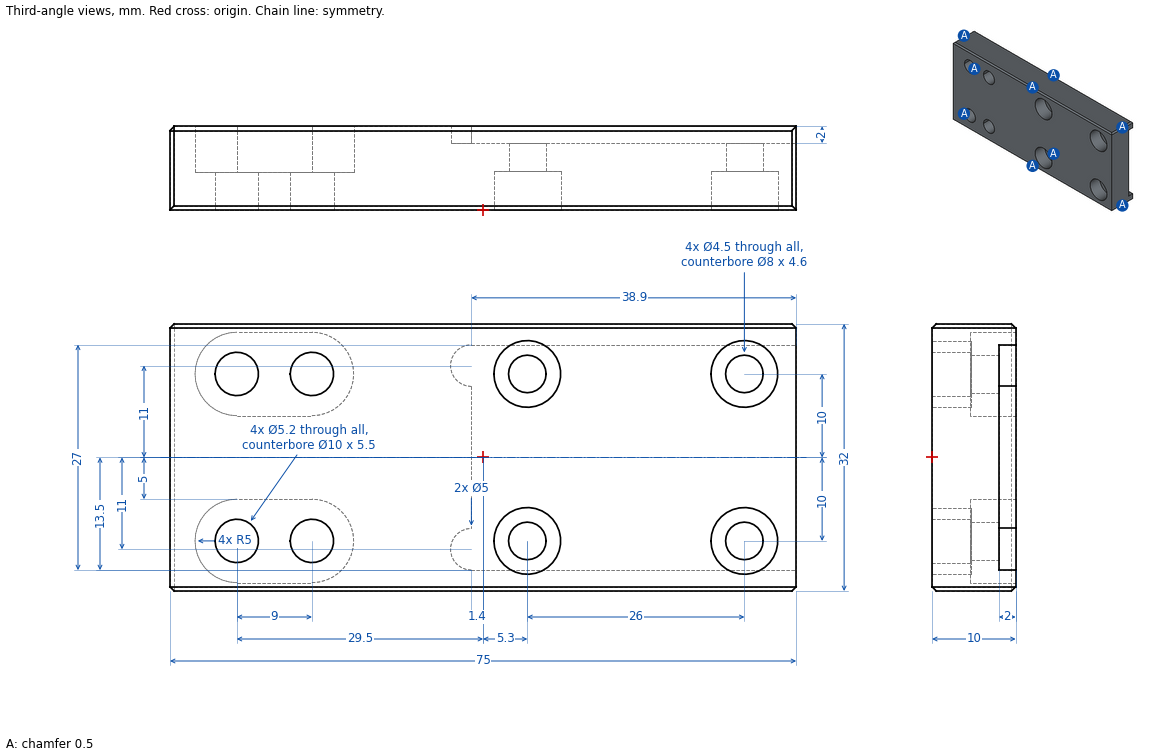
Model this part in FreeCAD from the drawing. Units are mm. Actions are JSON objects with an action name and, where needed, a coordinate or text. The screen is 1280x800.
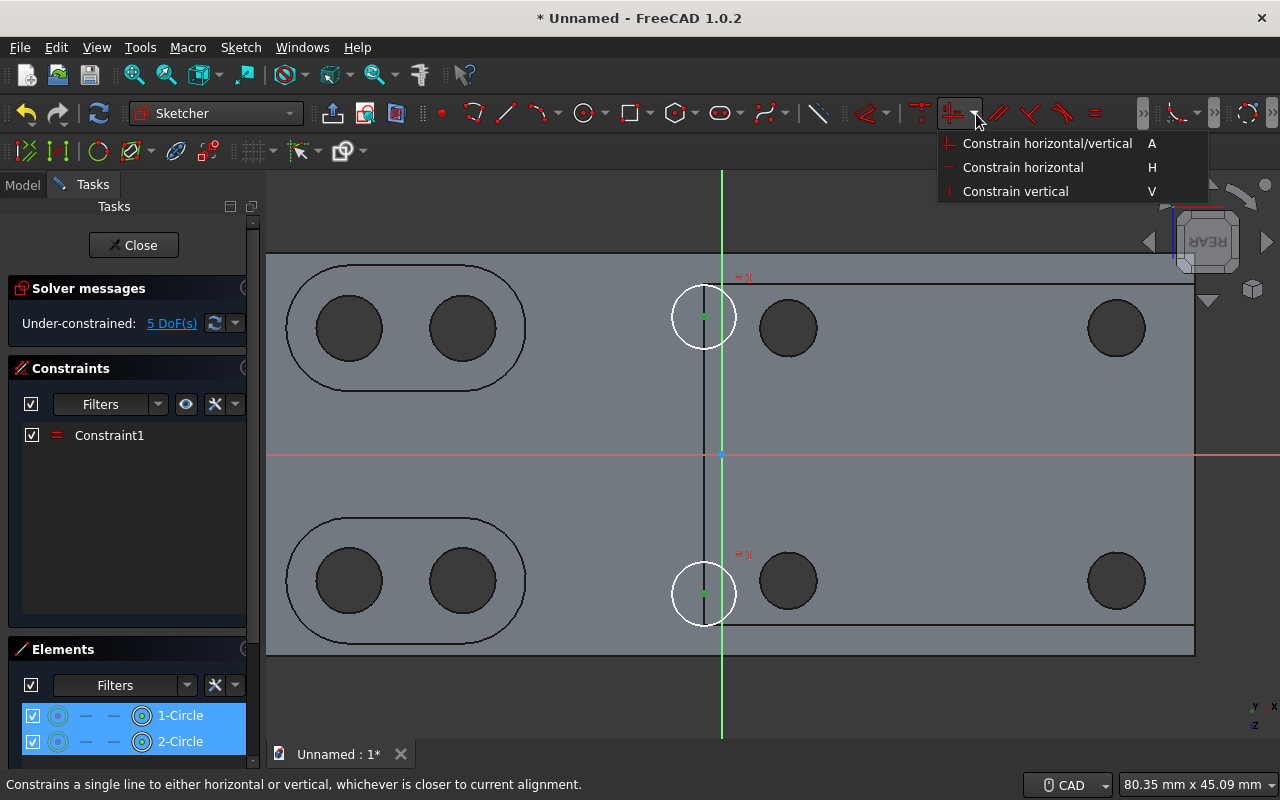
{"action": "left_click", "coordinate": [1073, 191]}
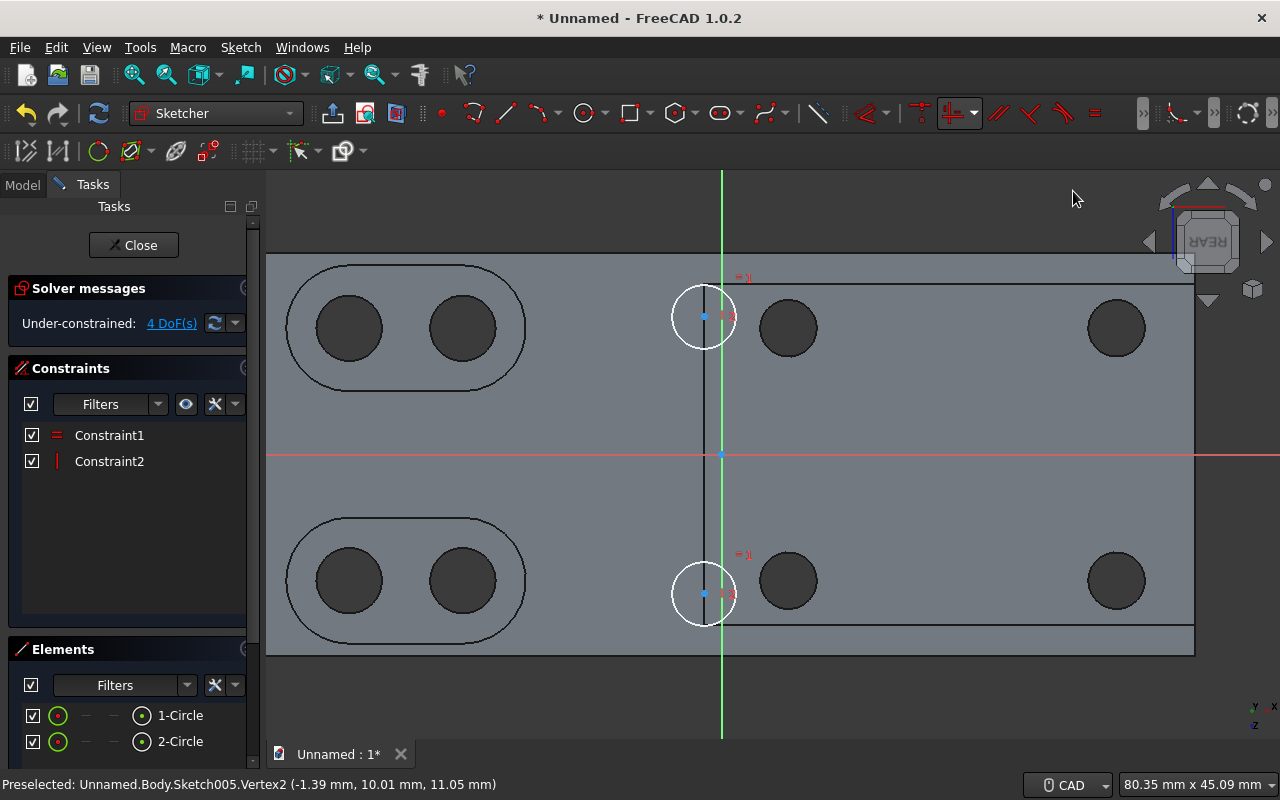
{"action": "left_click", "coordinate": [866, 114]}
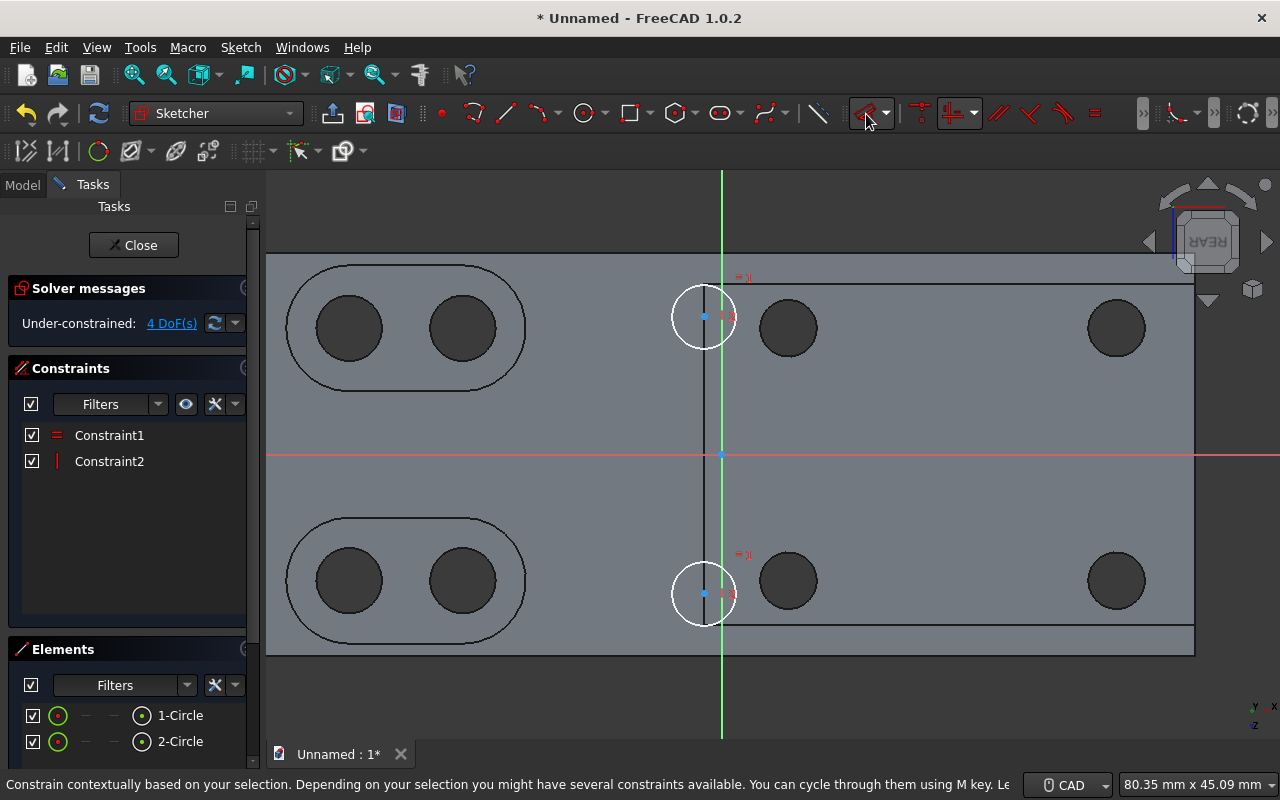
{"action": "left_click", "coordinate": [681, 295]}
{"action": "left_click", "coordinate": [658, 273]}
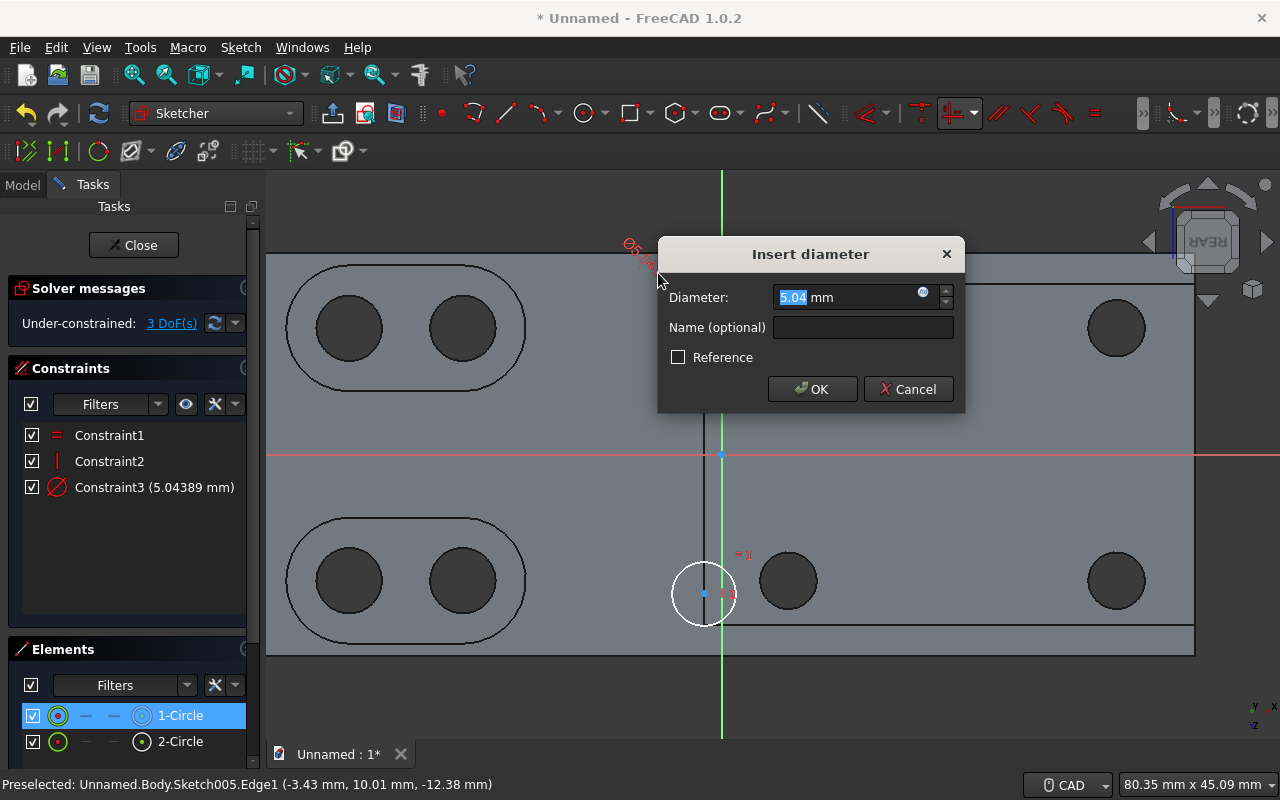
{"action": "type", "text": "5"}
{"action": "key", "text": "Return"}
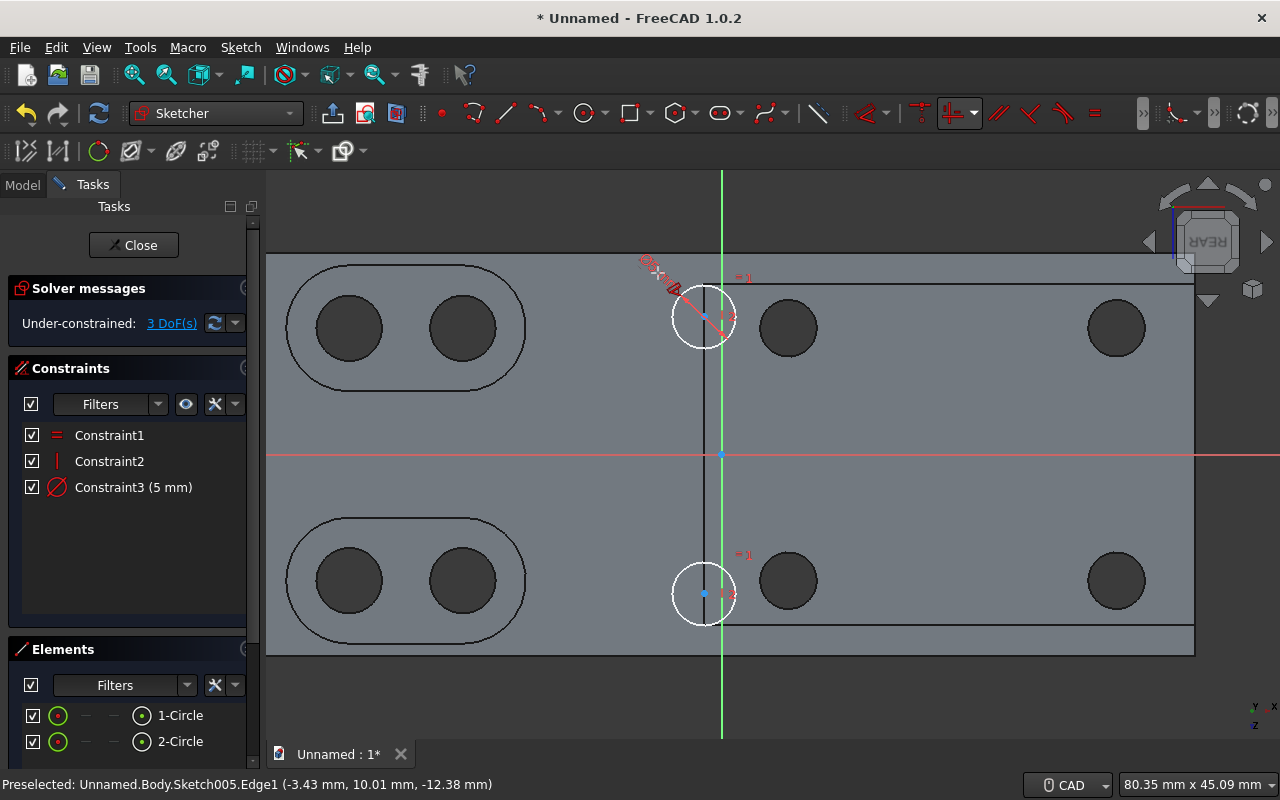
{"action": "left_click", "coordinate": [704, 317]}
{"action": "left_click", "coordinate": [756, 386]}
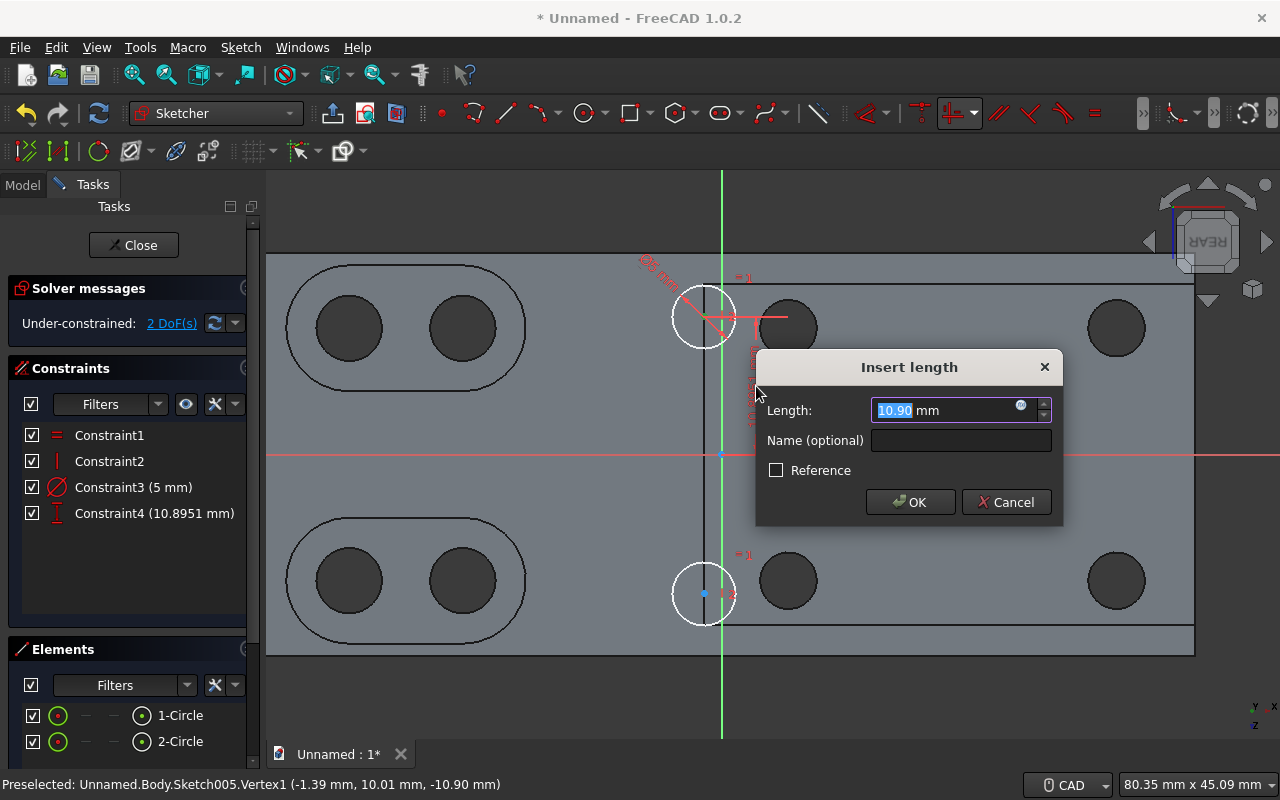
{"action": "type", "text": "11"}
{"action": "key", "text": "Return"}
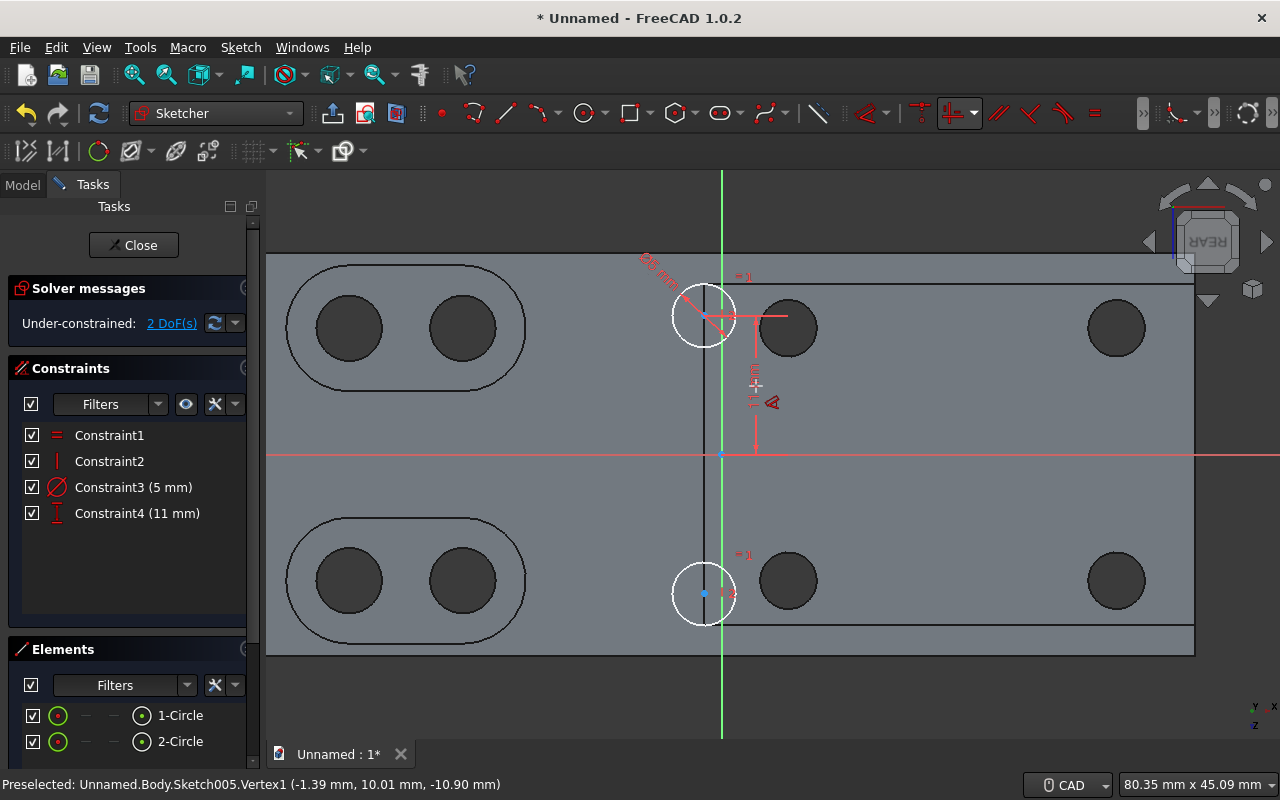
{"action": "left_click", "coordinate": [704, 594]}
{"action": "left_click", "coordinate": [756, 524]}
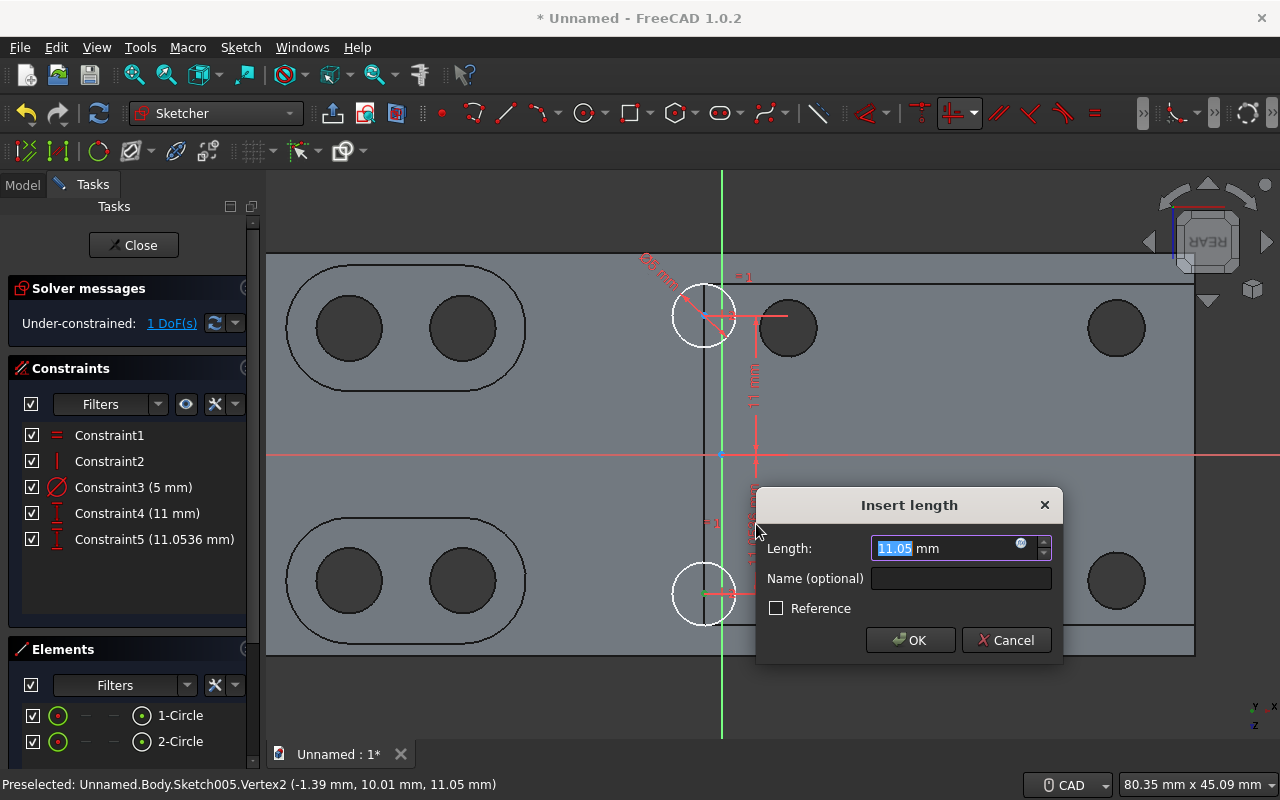
{"action": "type", "text": "11"}
{"action": "key", "text": "Return"}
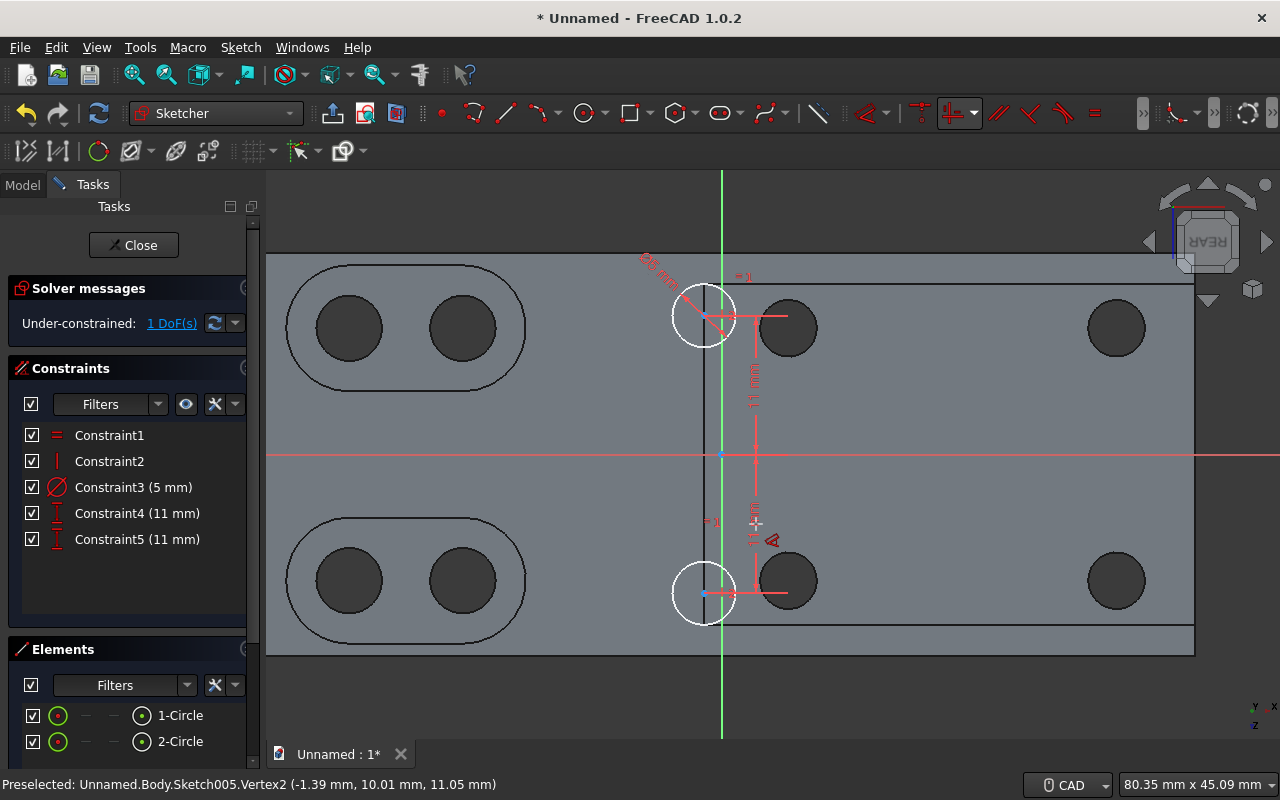
{"action": "scroll", "coordinate": [704, 316], "scroll_direction": "up", "scroll_amount": 5}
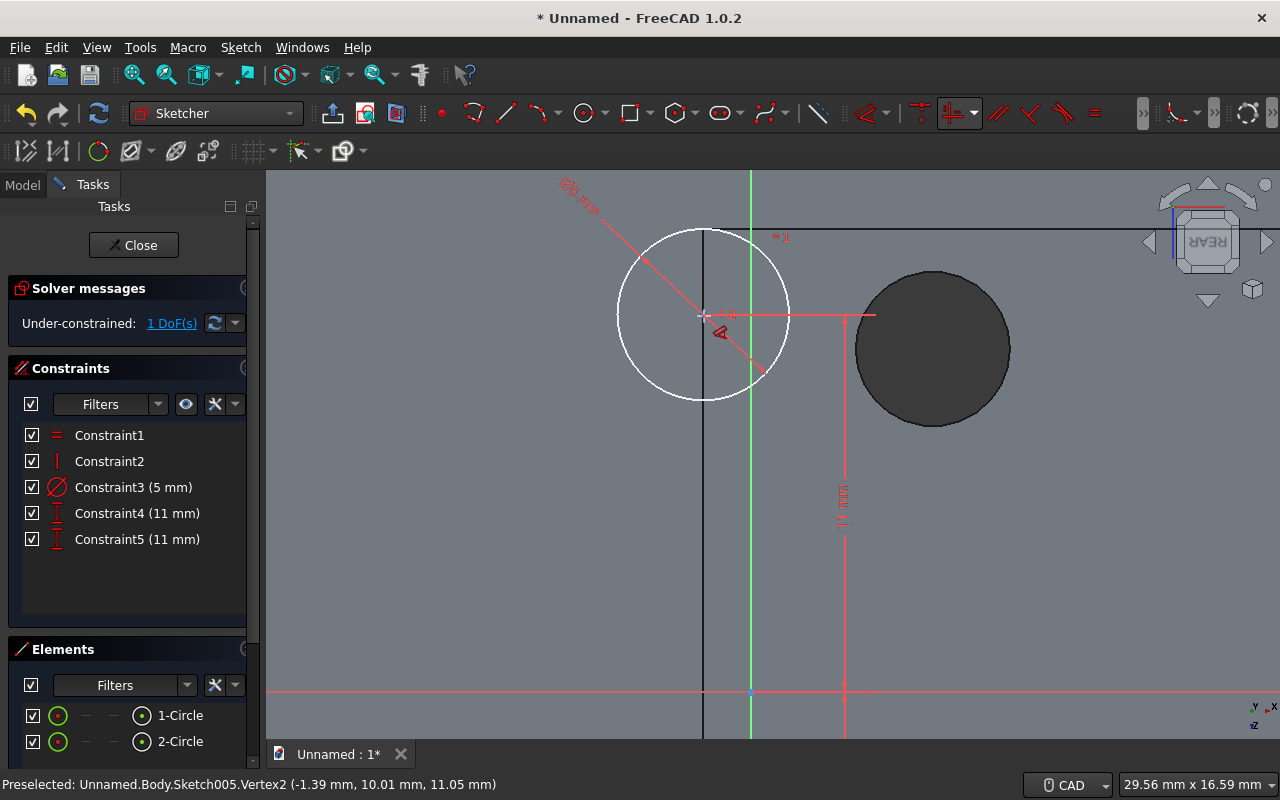
{"action": "left_click", "coordinate": [703, 315]}
{"action": "left_click", "coordinate": [727, 281]}